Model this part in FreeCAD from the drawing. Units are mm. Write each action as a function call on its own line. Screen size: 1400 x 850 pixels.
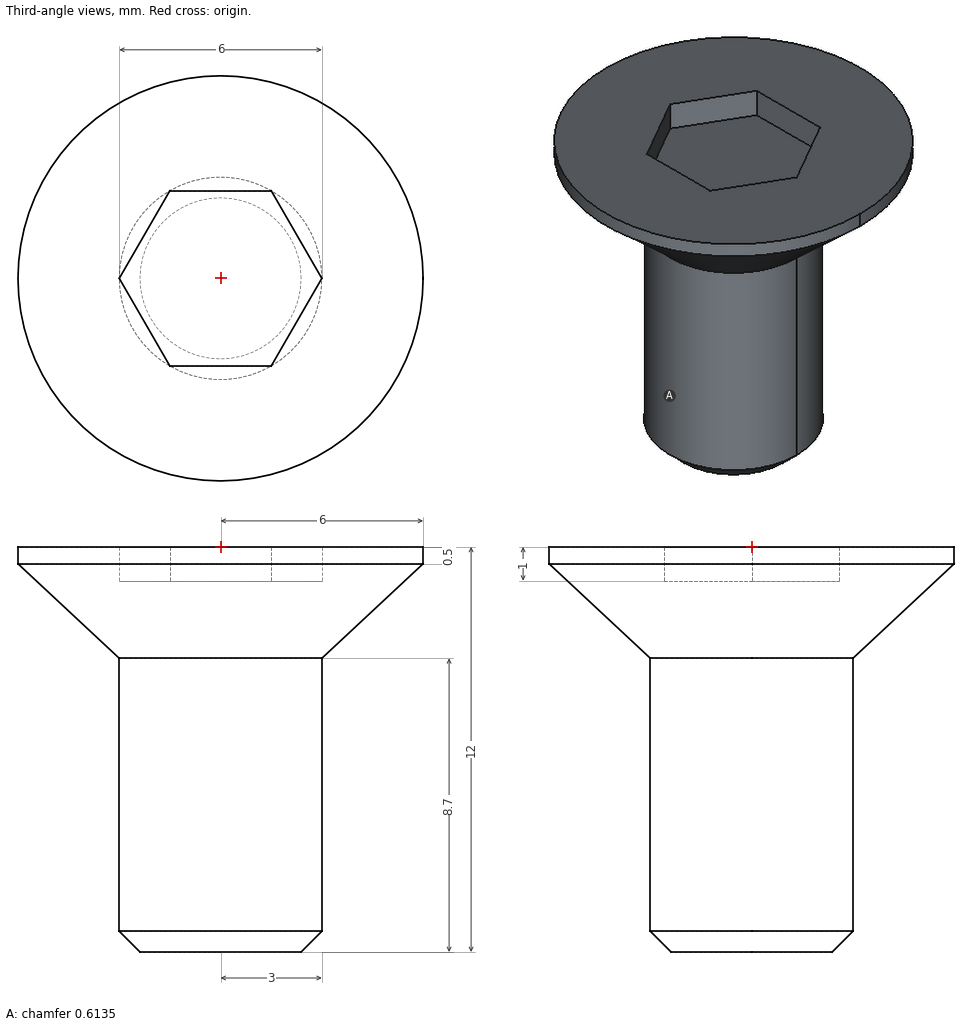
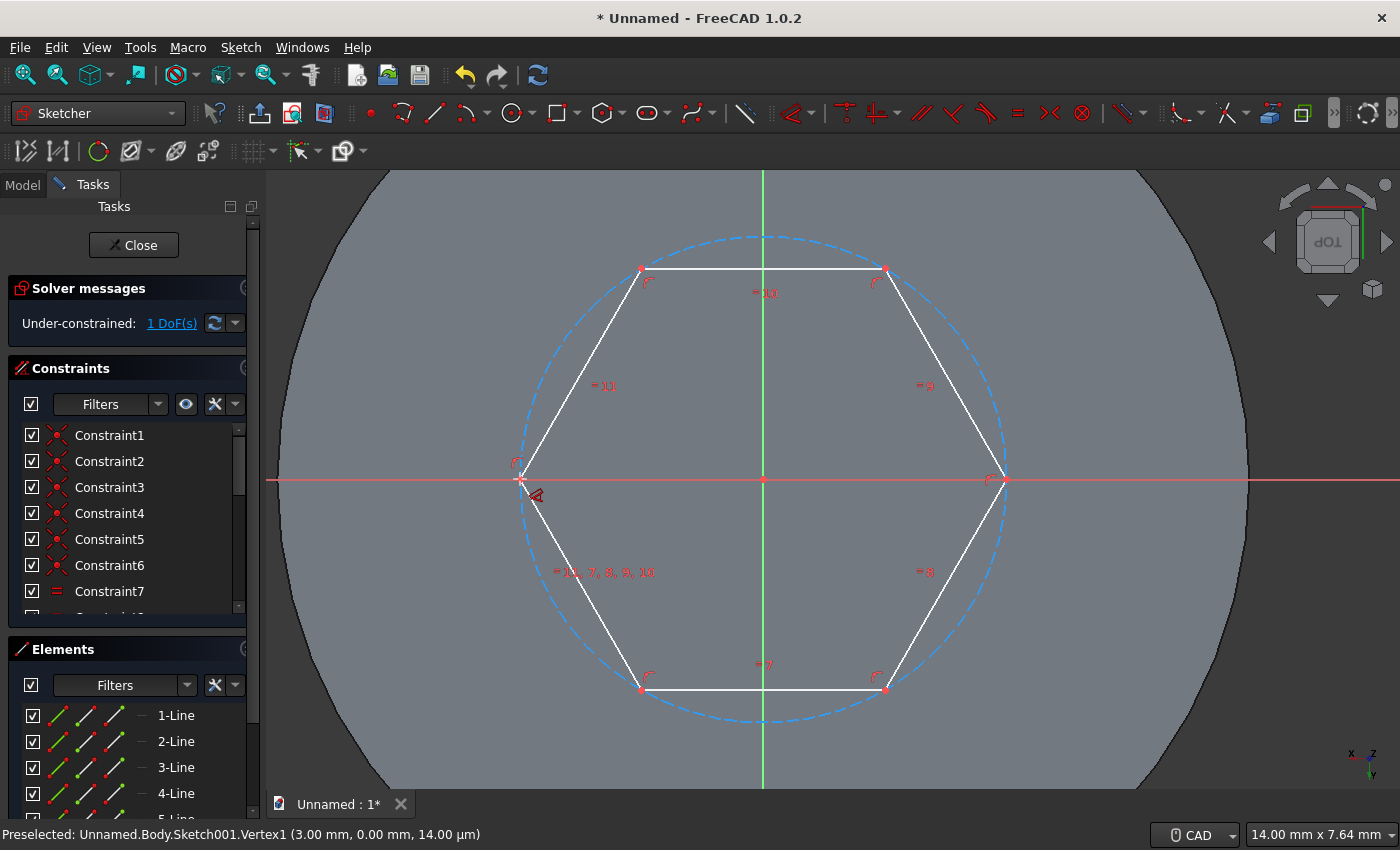
click(520, 479)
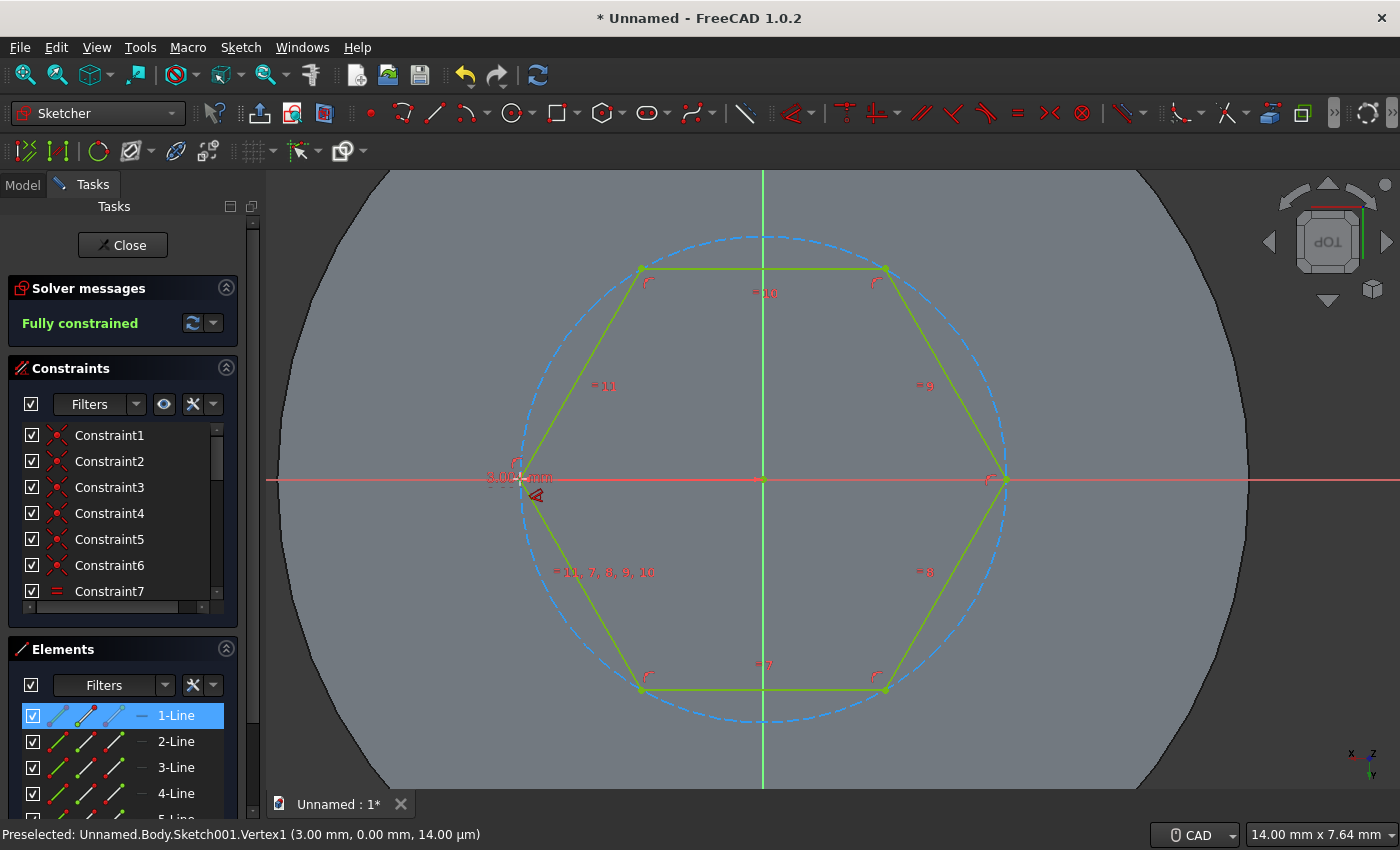
click(1007, 479)
click(651, 513)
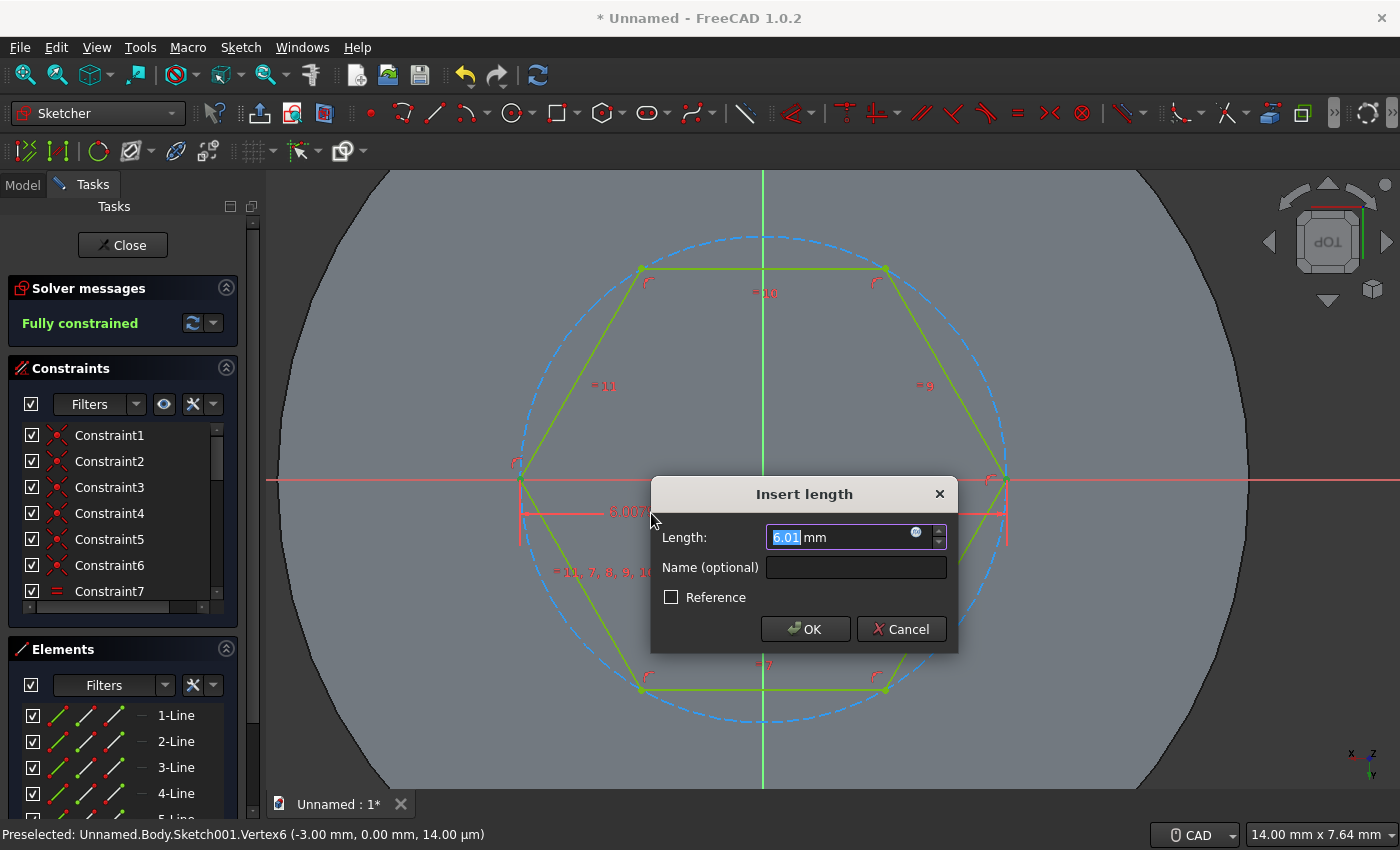
text(6)
key(Return)
key(Escape)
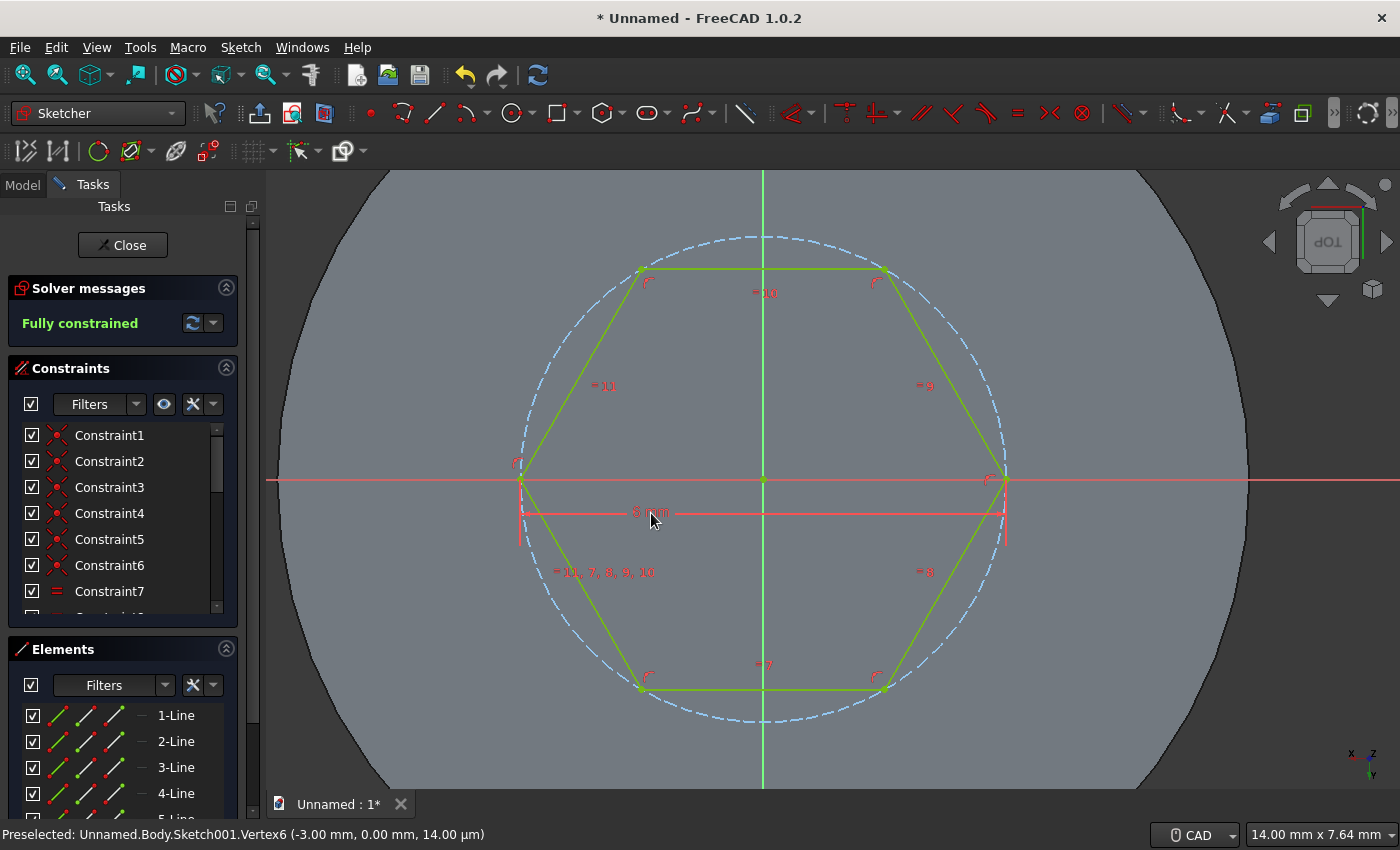
click(123, 245)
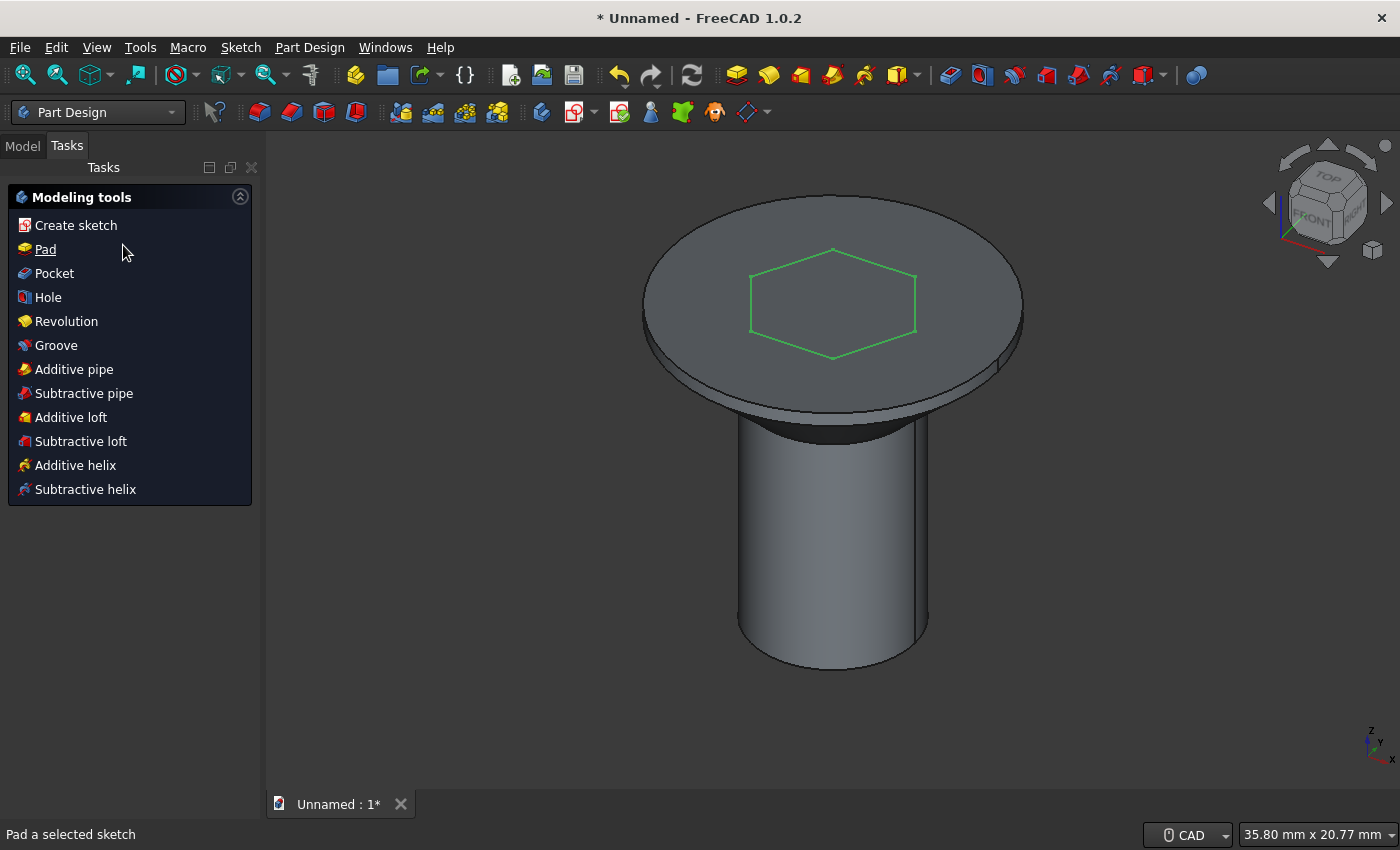
click(952, 76)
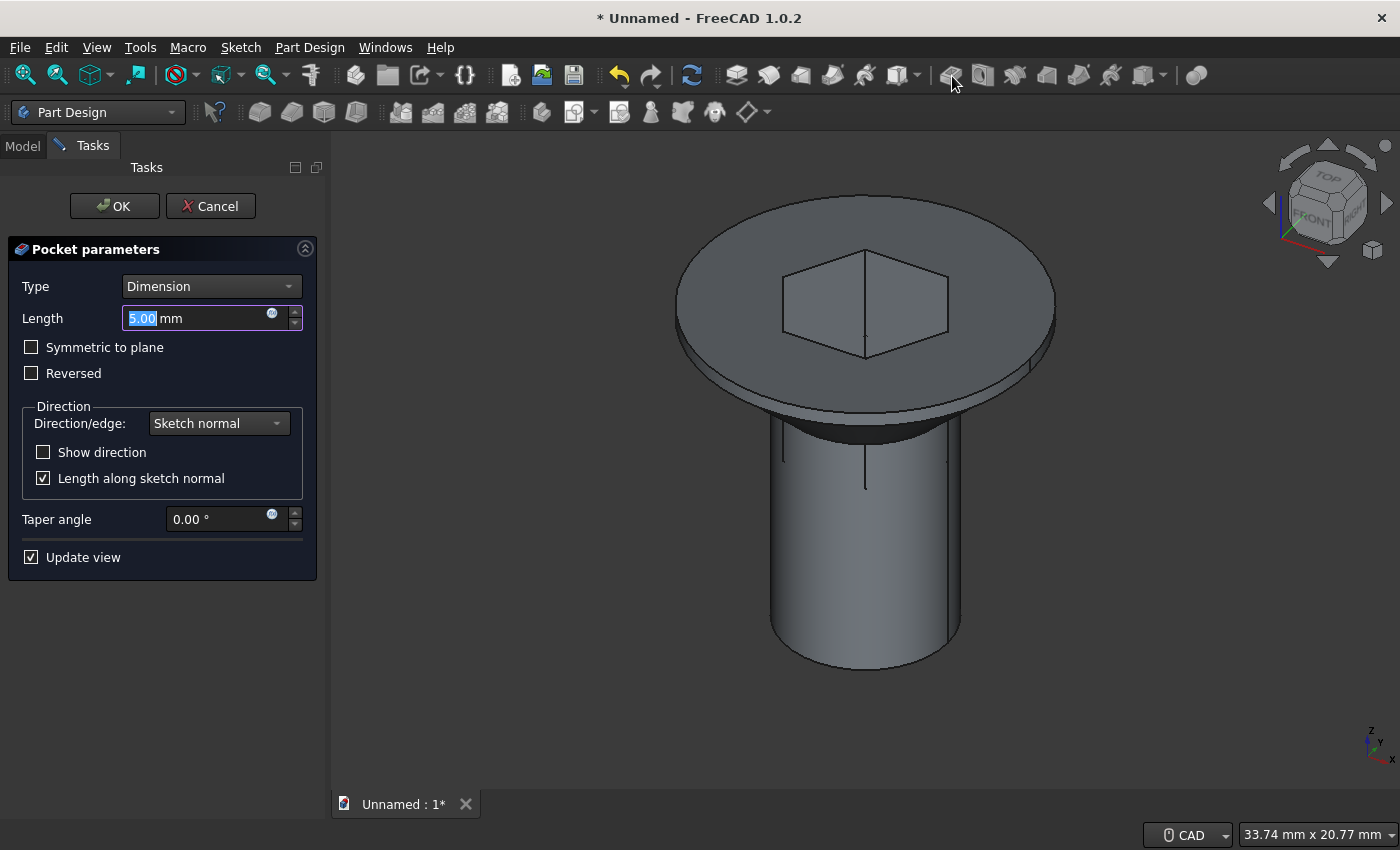
text(1)
key(Tab)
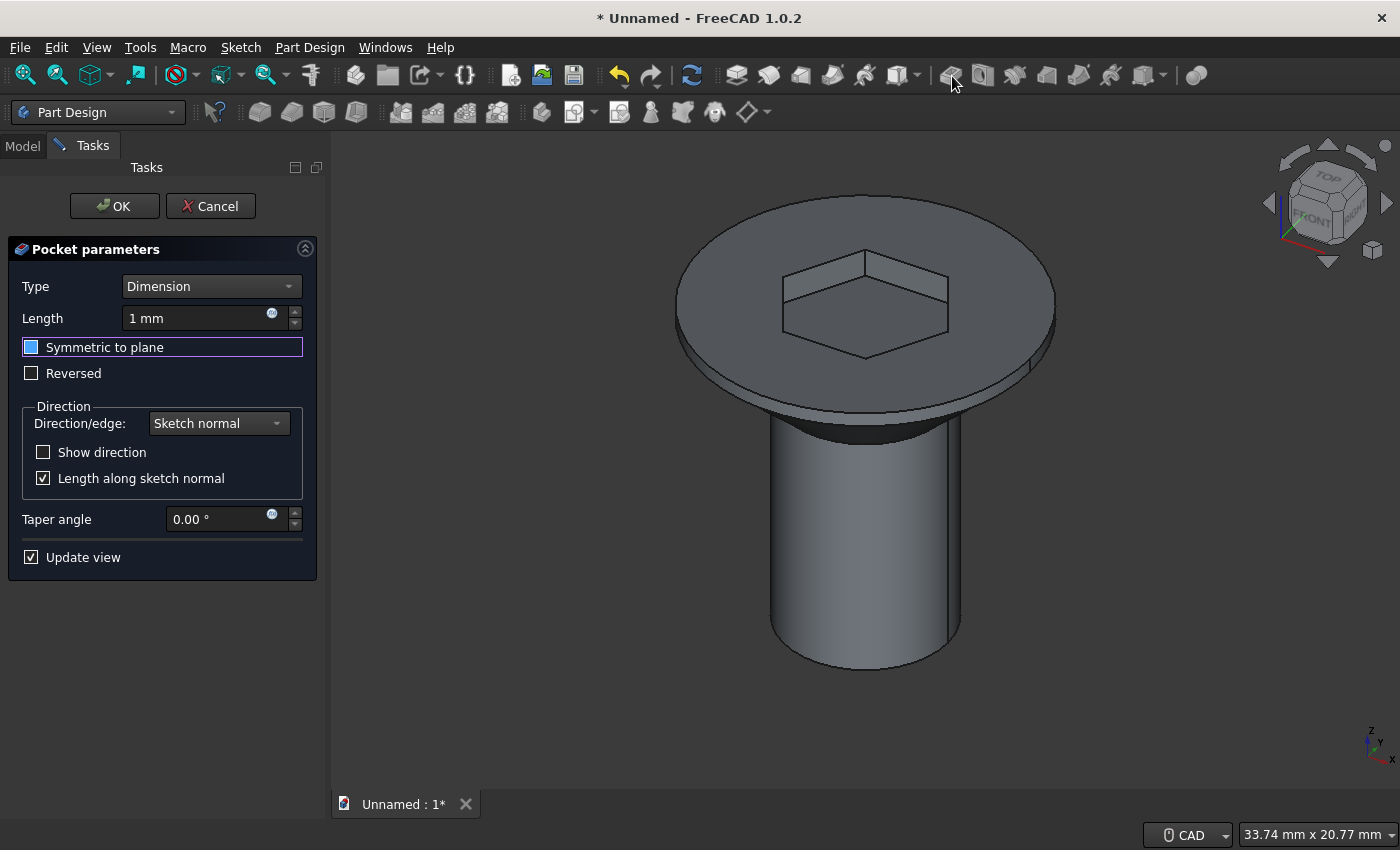
click(115, 206)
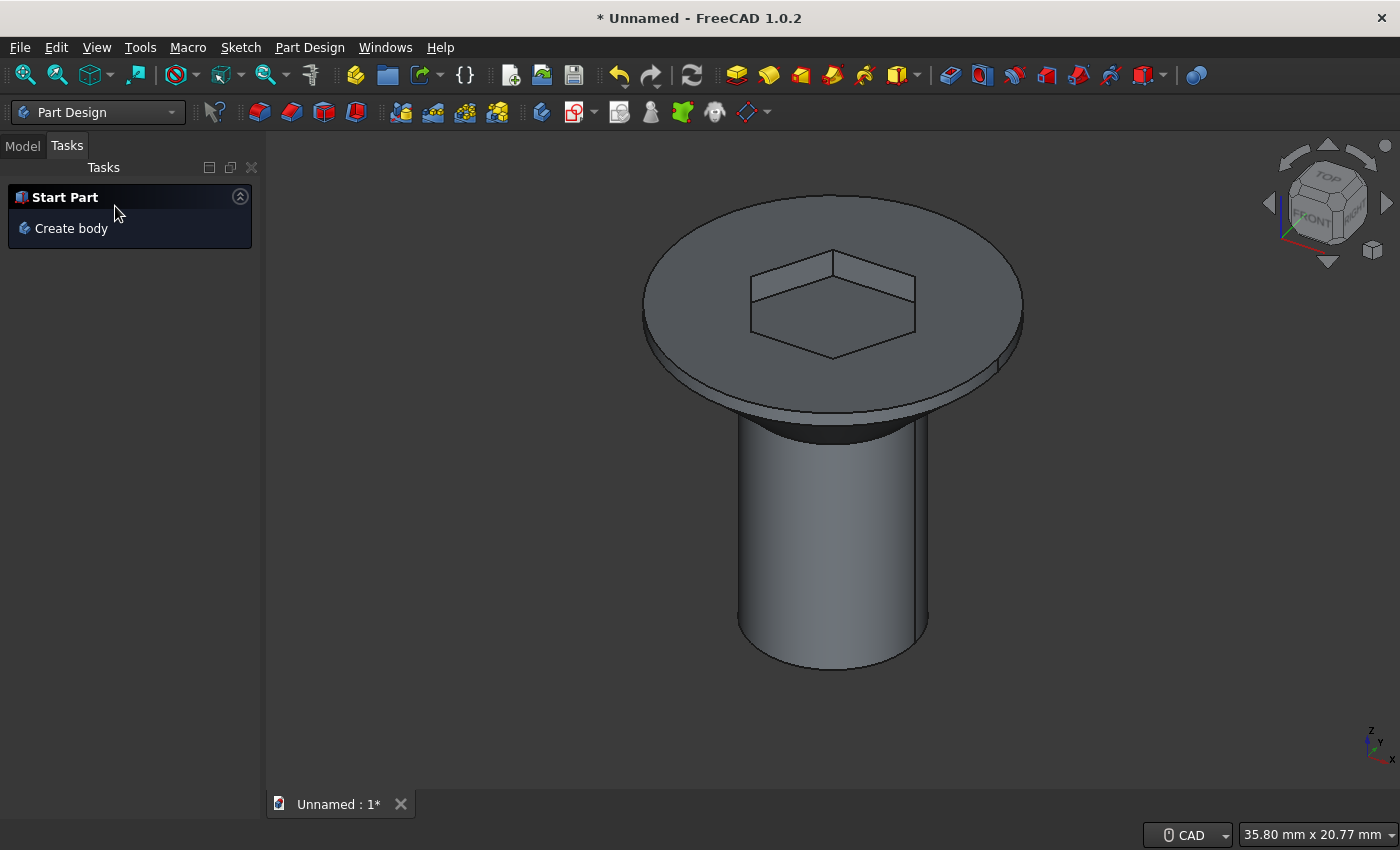
key(0)